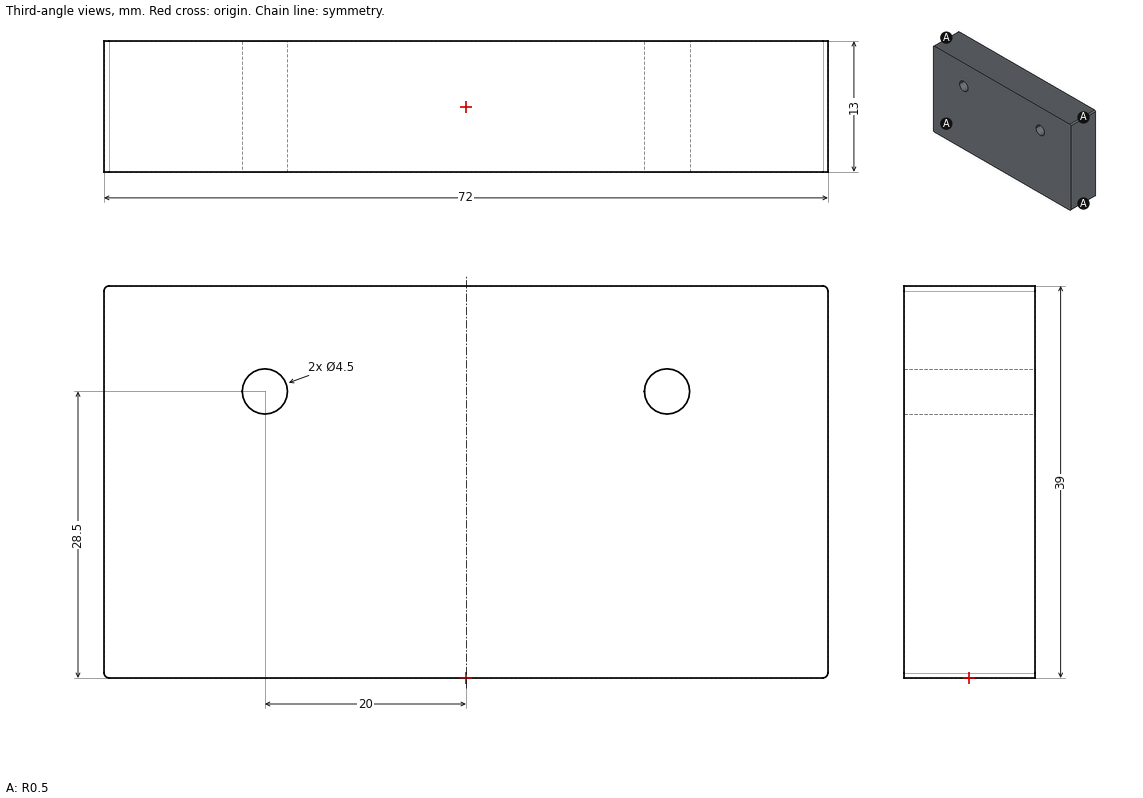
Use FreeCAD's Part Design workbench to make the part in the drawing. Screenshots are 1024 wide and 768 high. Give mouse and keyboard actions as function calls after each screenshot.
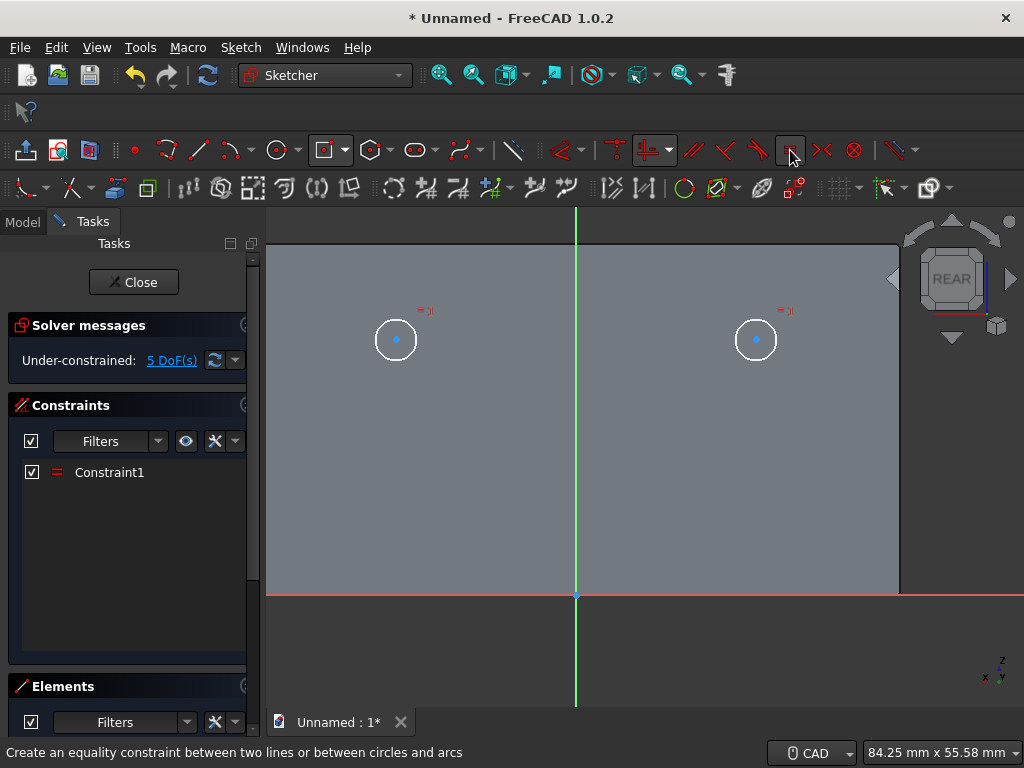
click(756, 340)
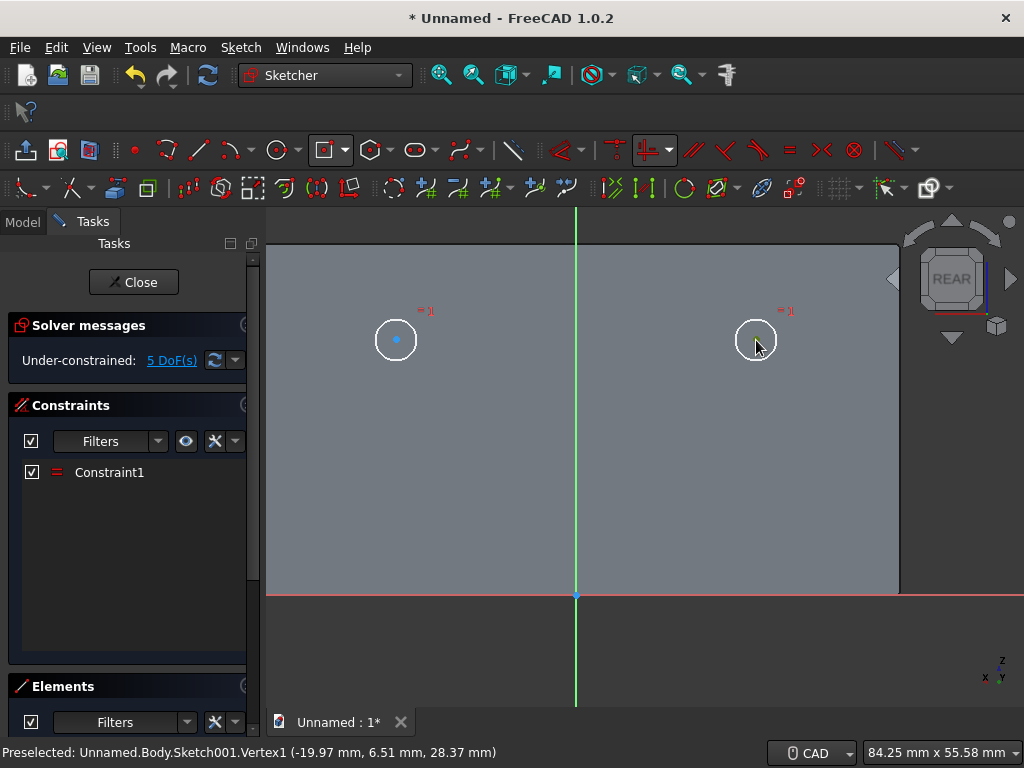
click(396, 340)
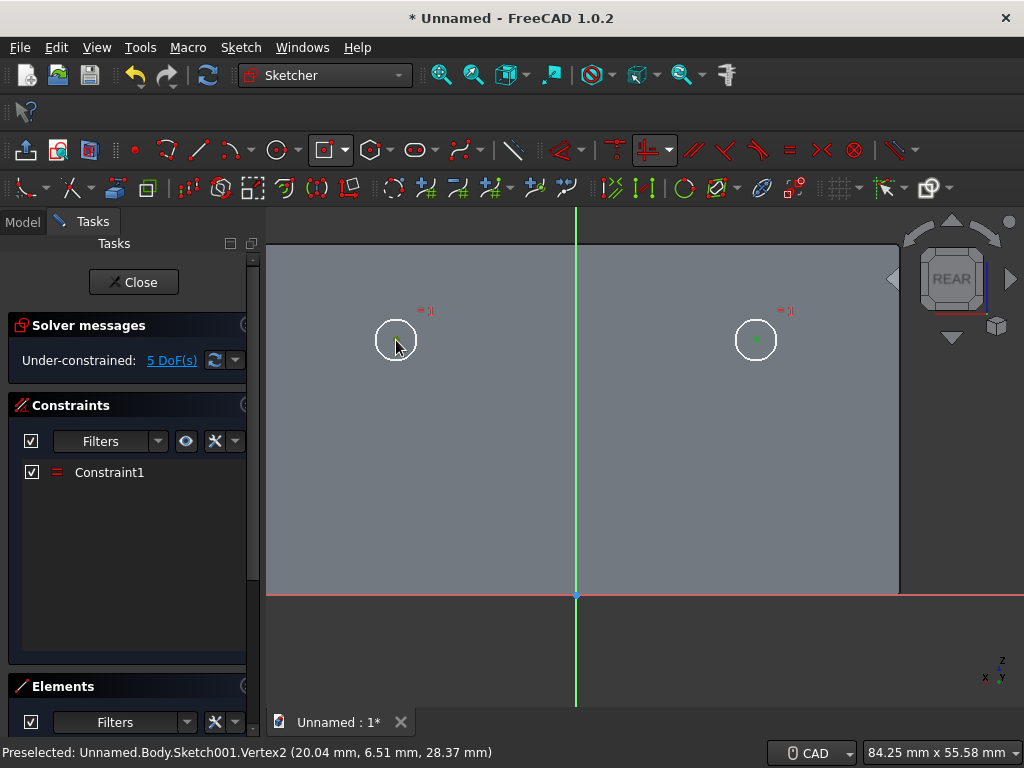
click(576, 647)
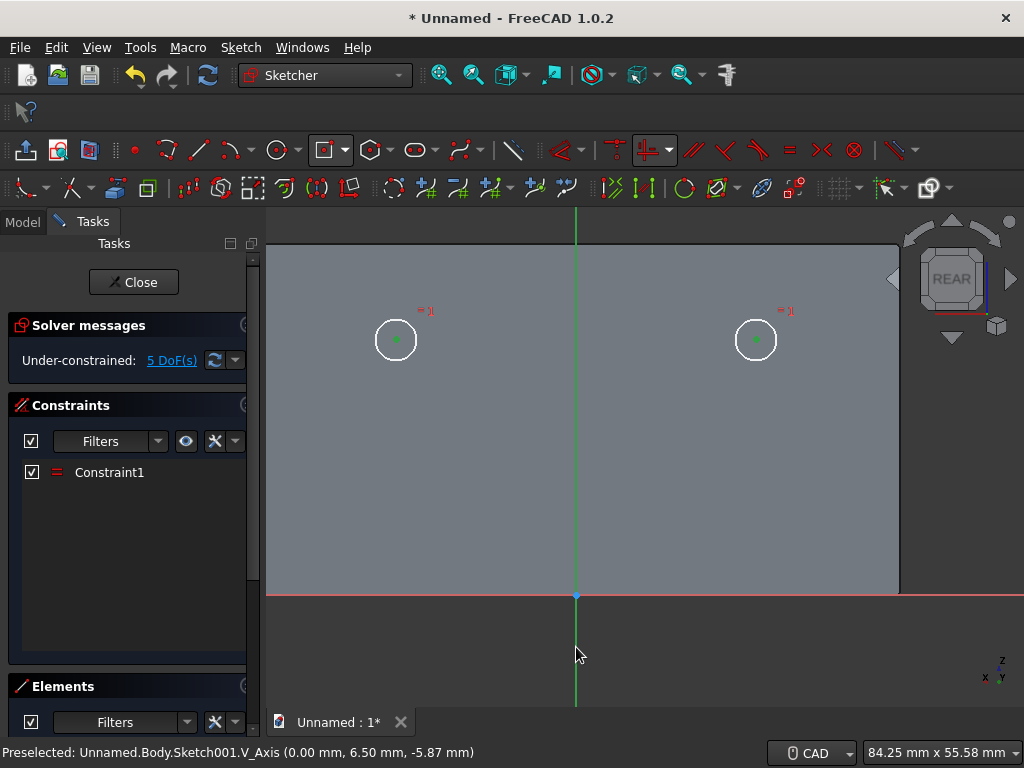
click(822, 150)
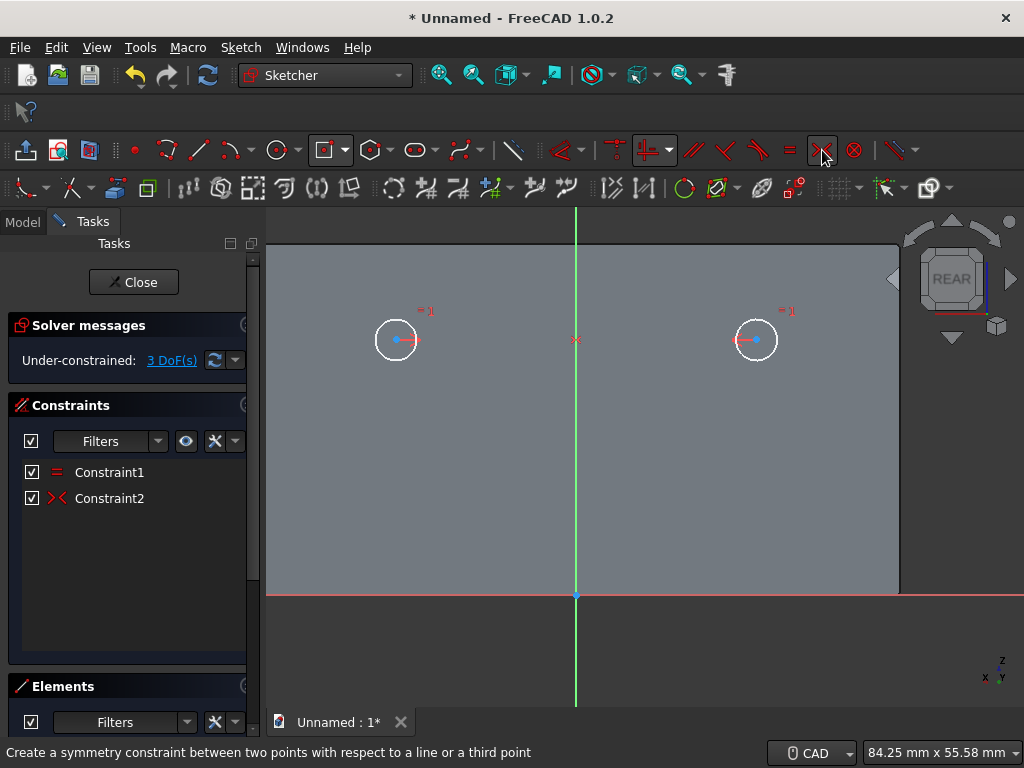
click(560, 150)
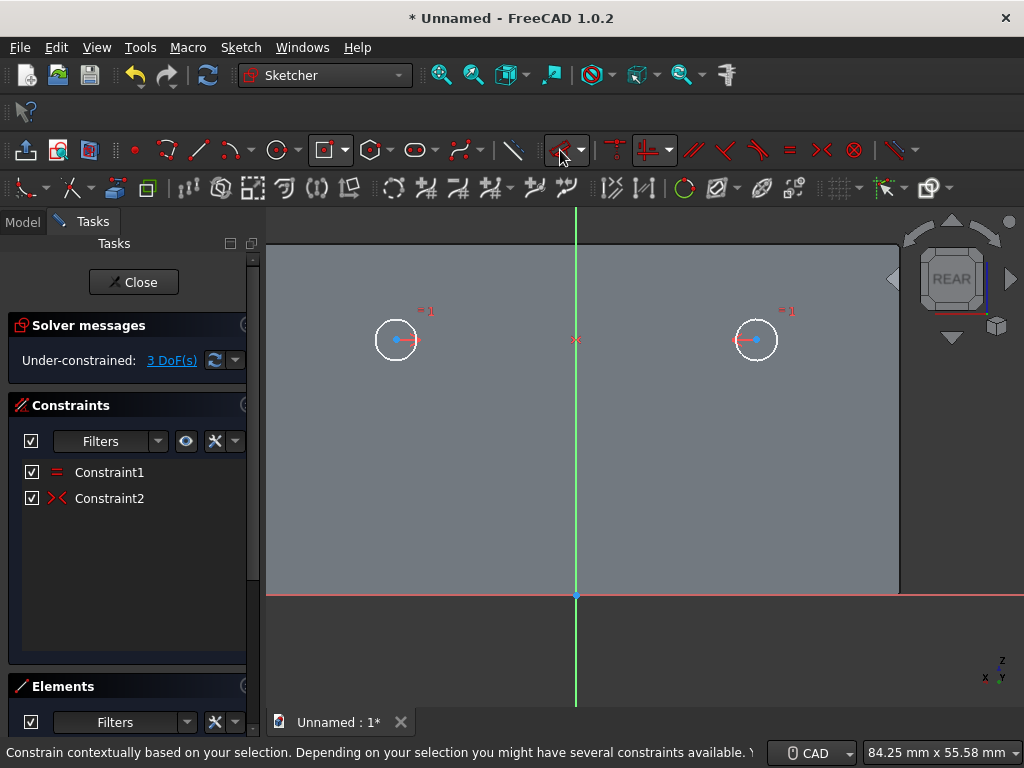
click(771, 325)
click(793, 302)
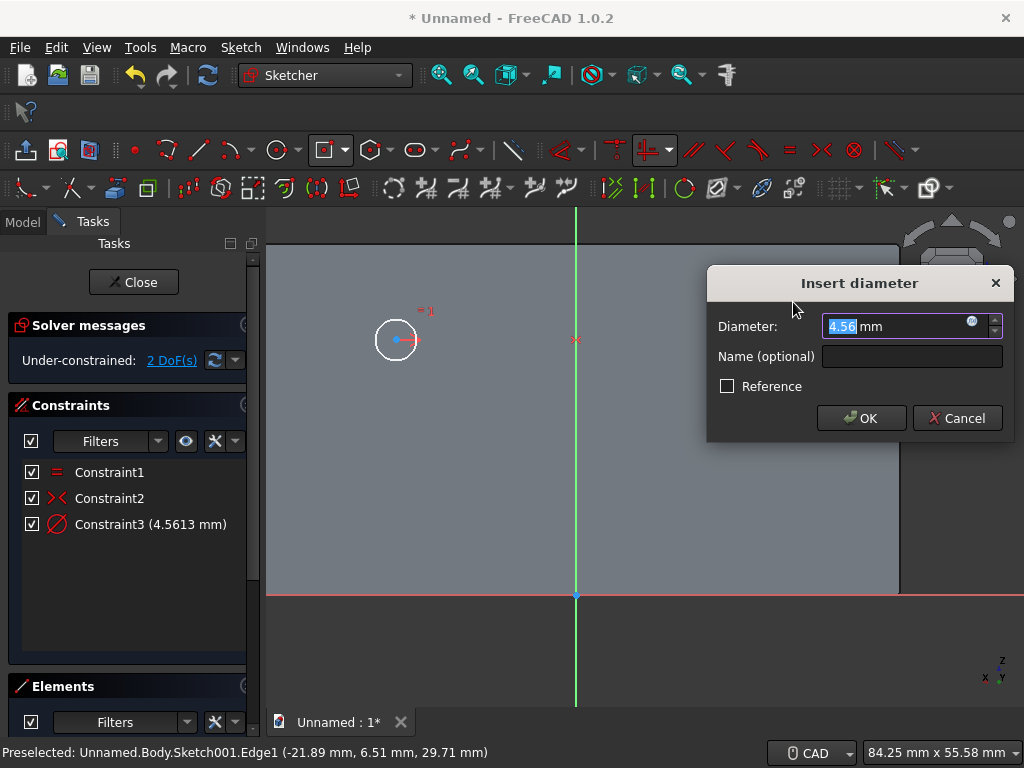
text(4.5)
key(Return)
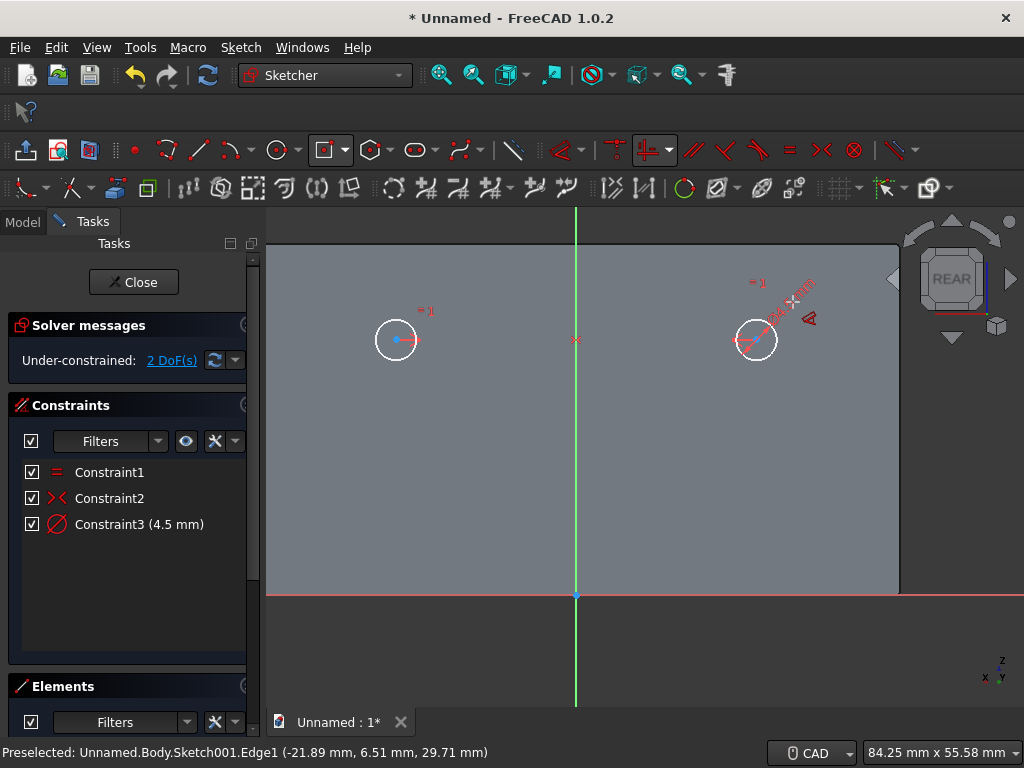
click(757, 340)
click(666, 629)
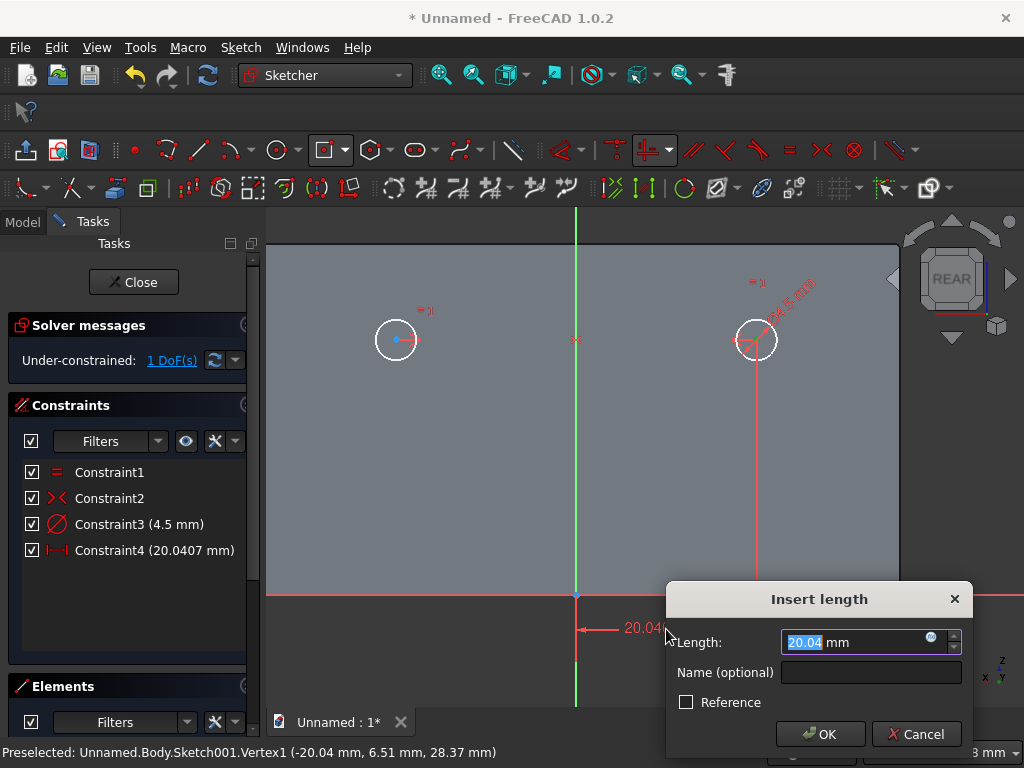
text(20)
key(Return)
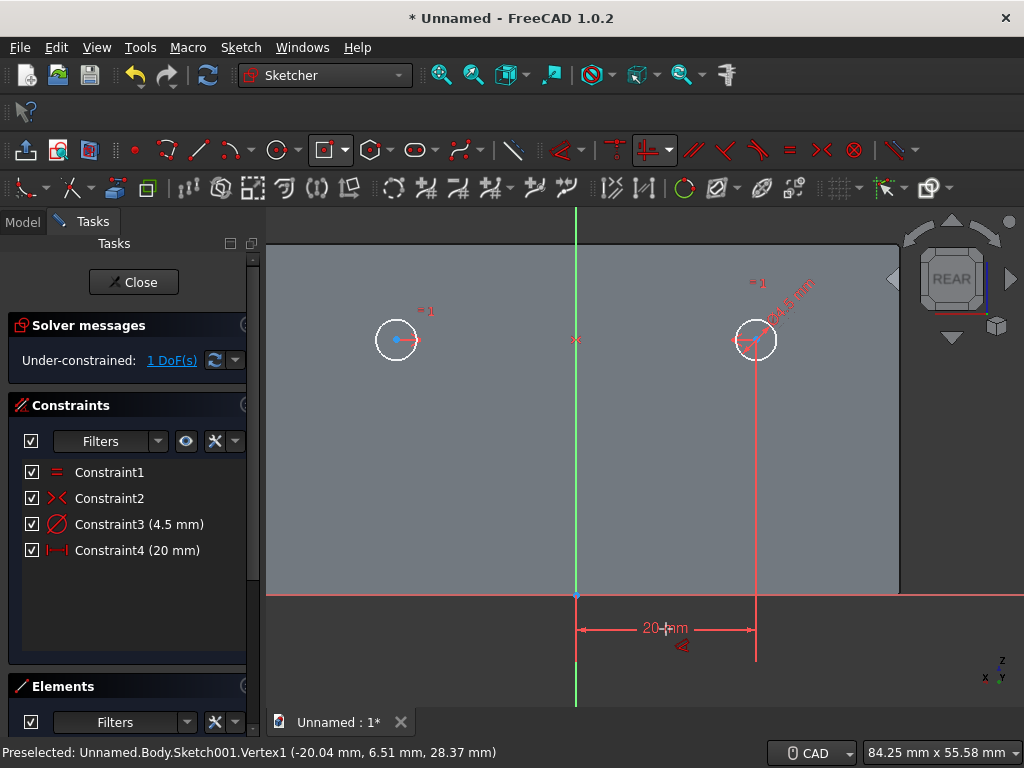
click(756, 340)
click(790, 468)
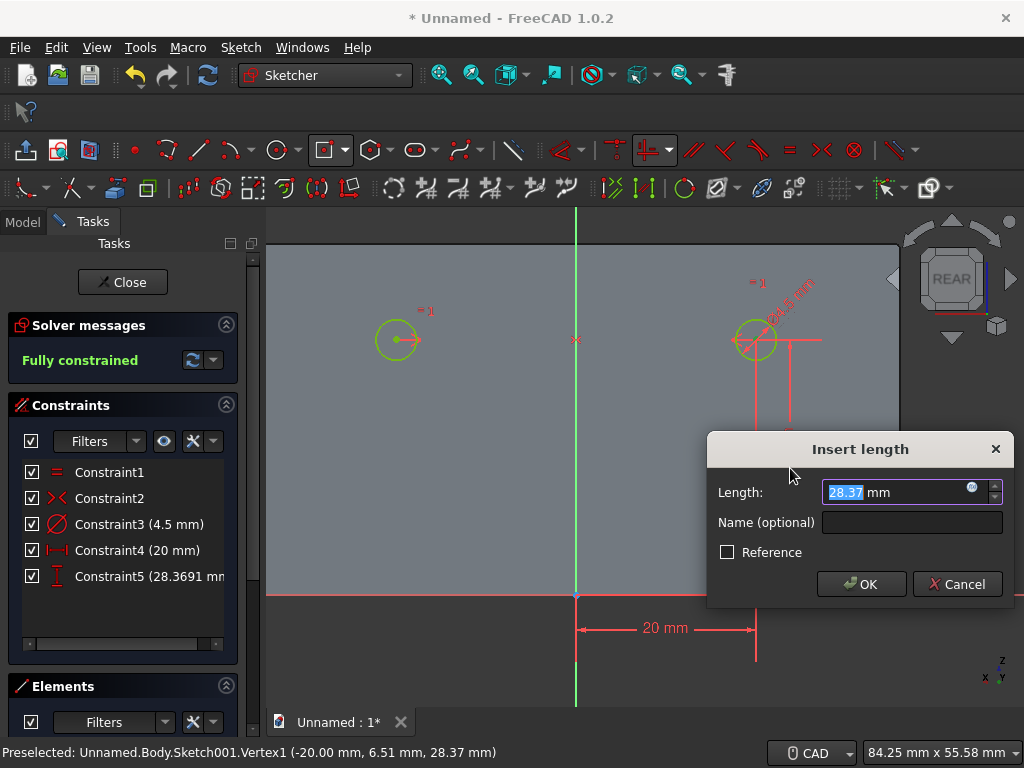
text(28.5)
key(Return)
key(Escape)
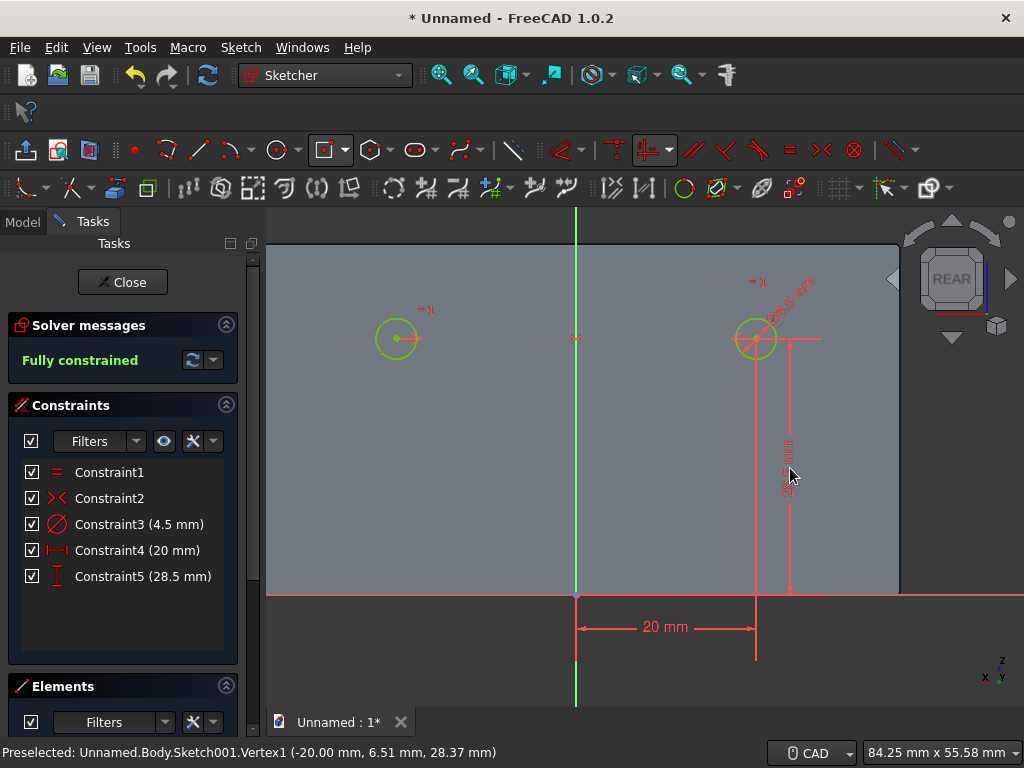
click(123, 282)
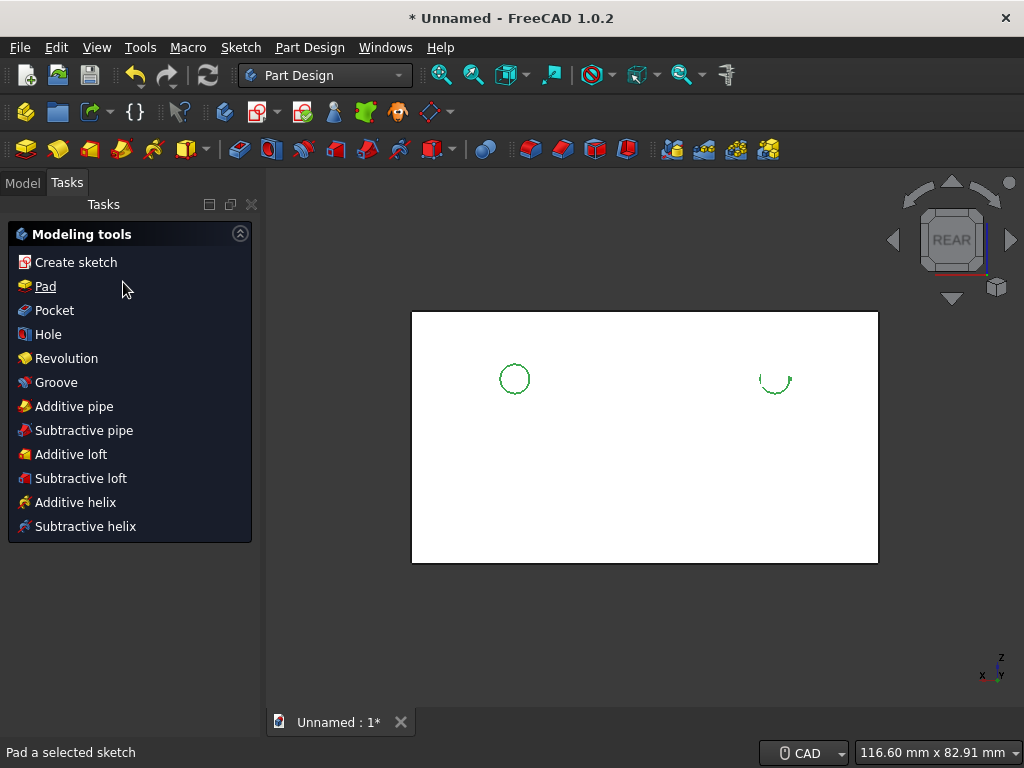
click(240, 150)